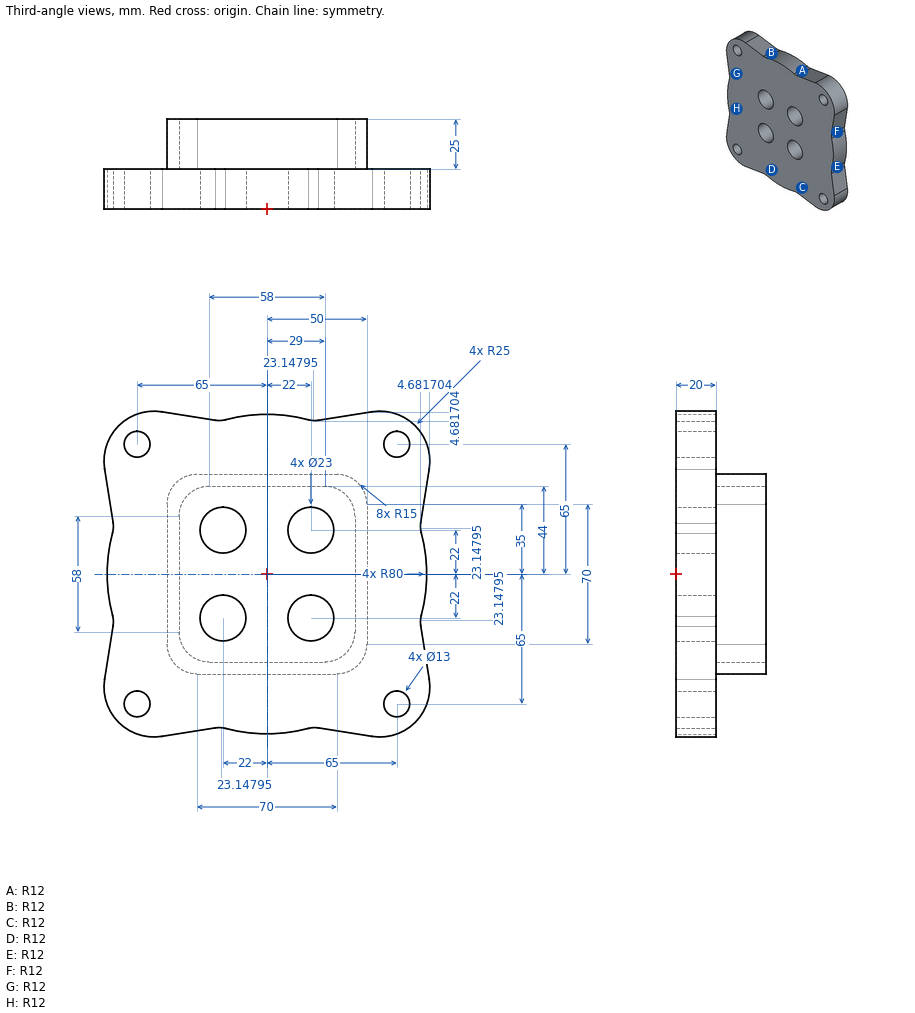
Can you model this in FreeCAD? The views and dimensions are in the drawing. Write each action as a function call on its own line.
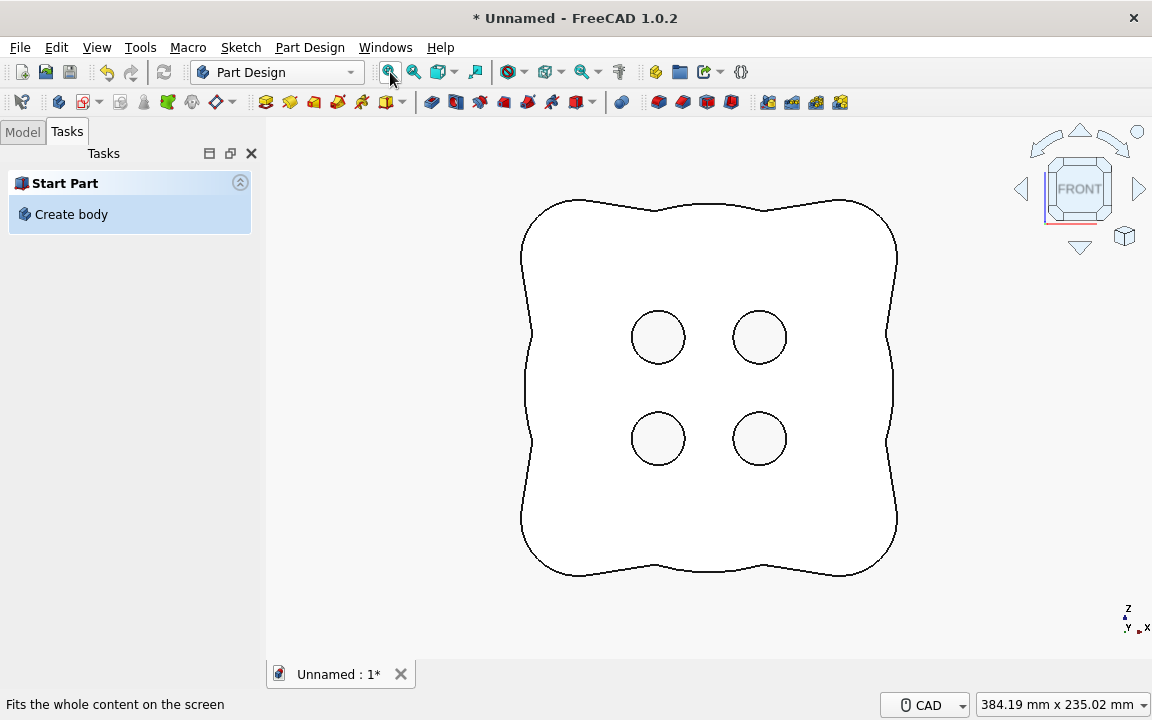
key(3)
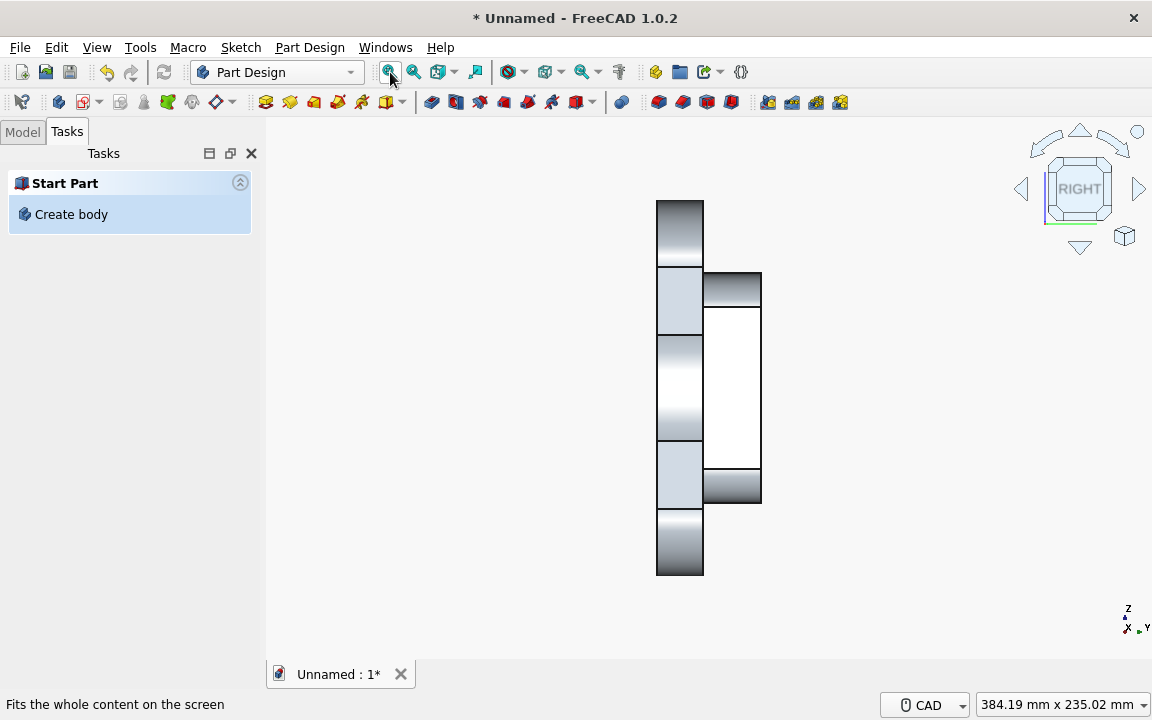
key(5)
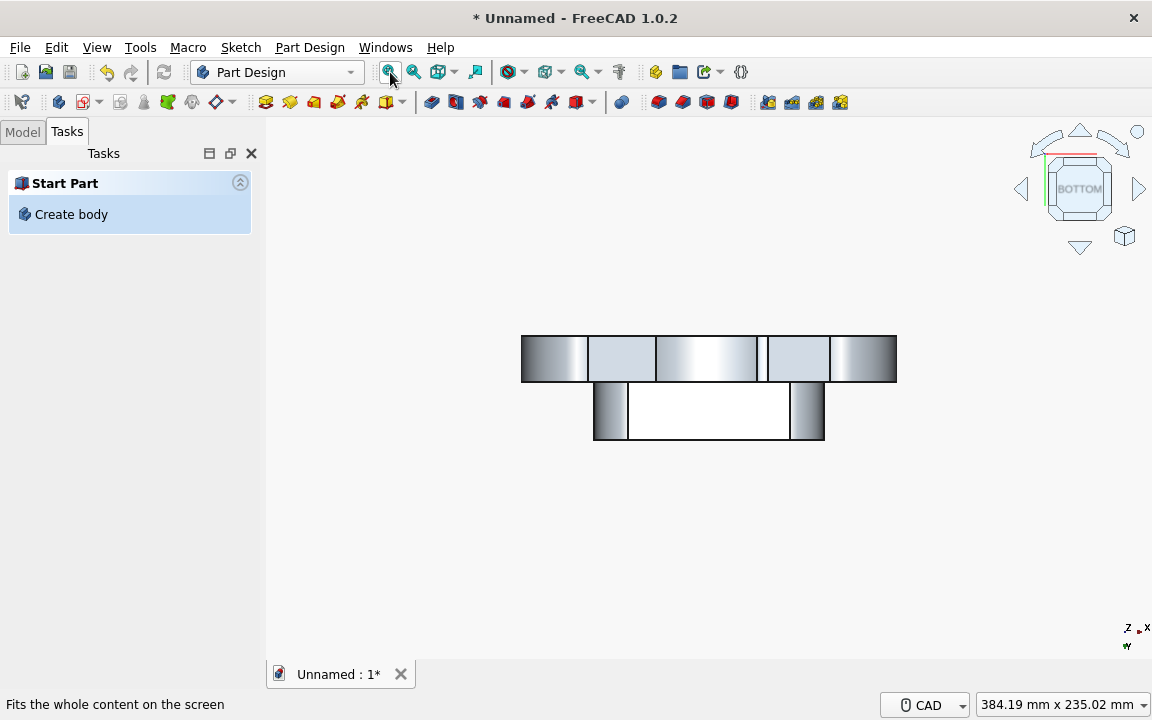
click(390, 72)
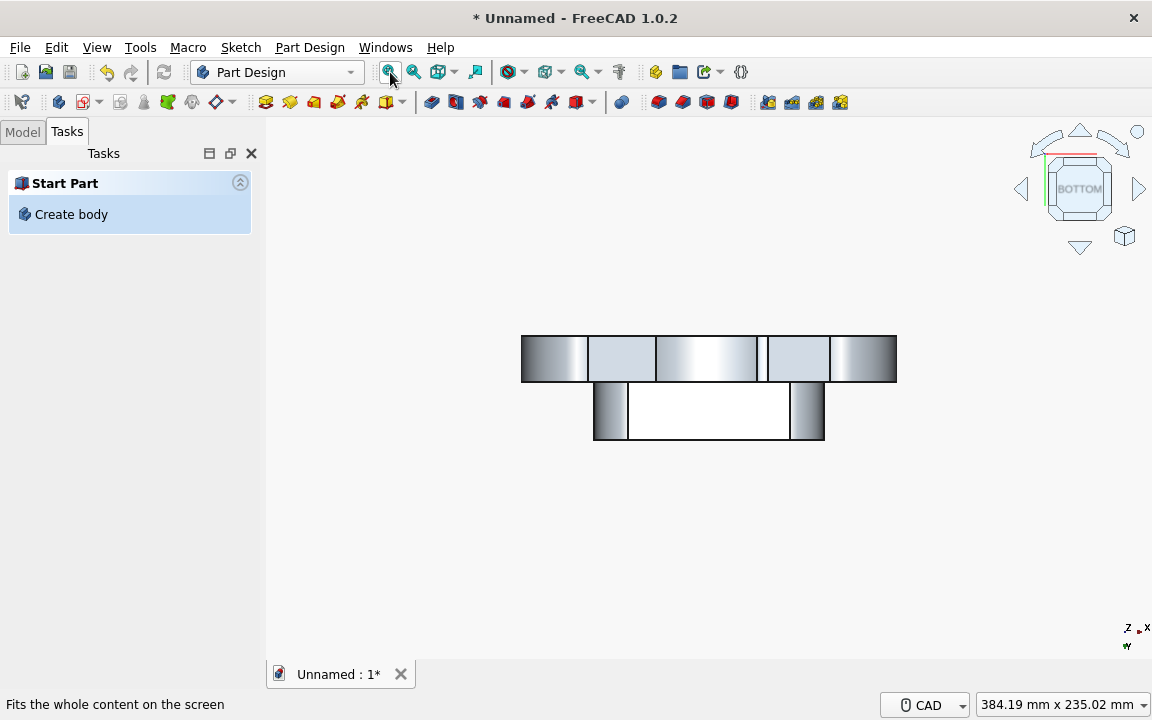
key(4)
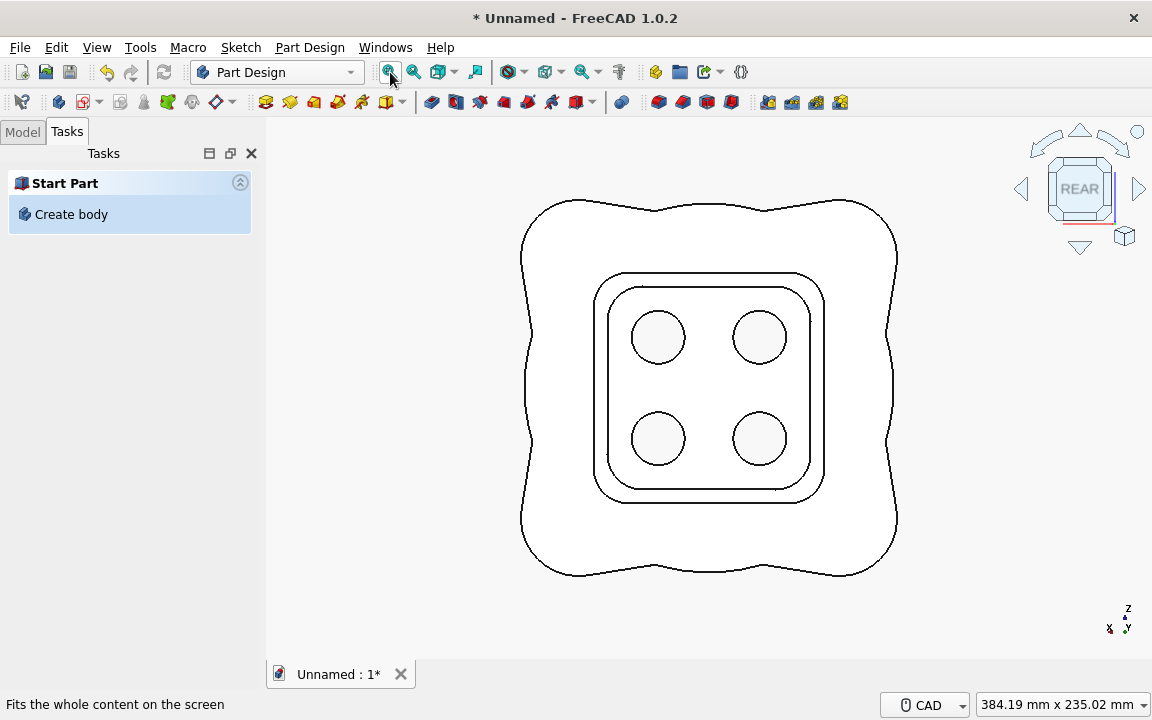
key(6)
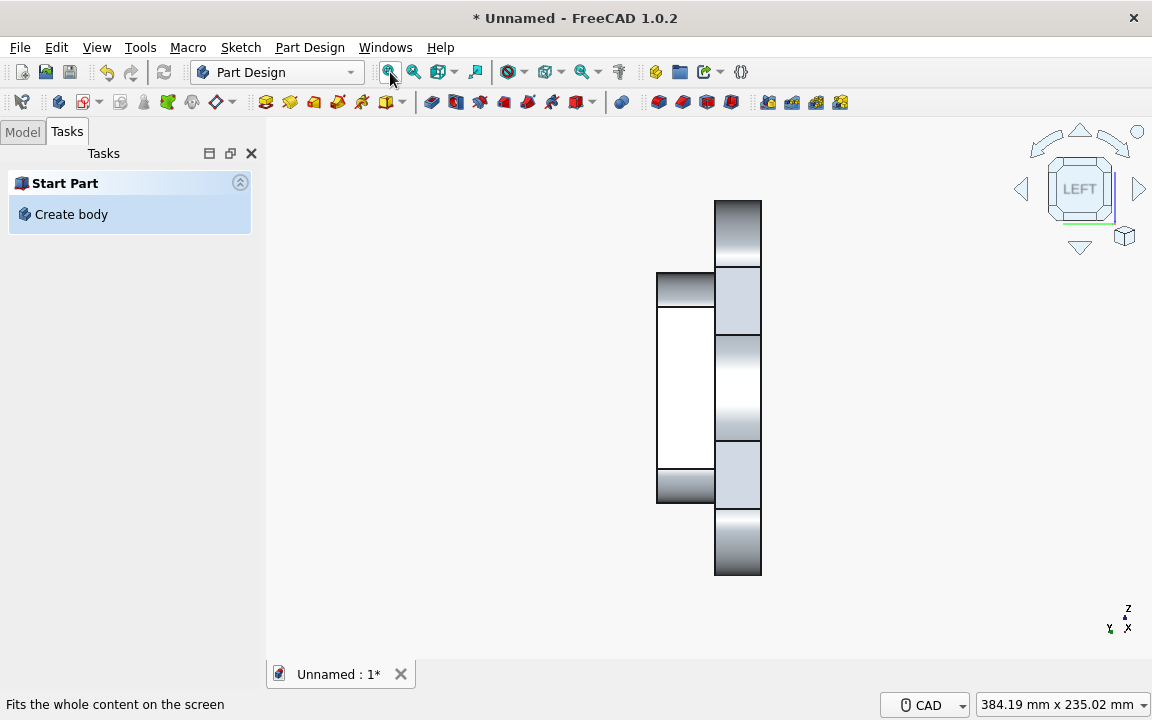
key(v)
key(3)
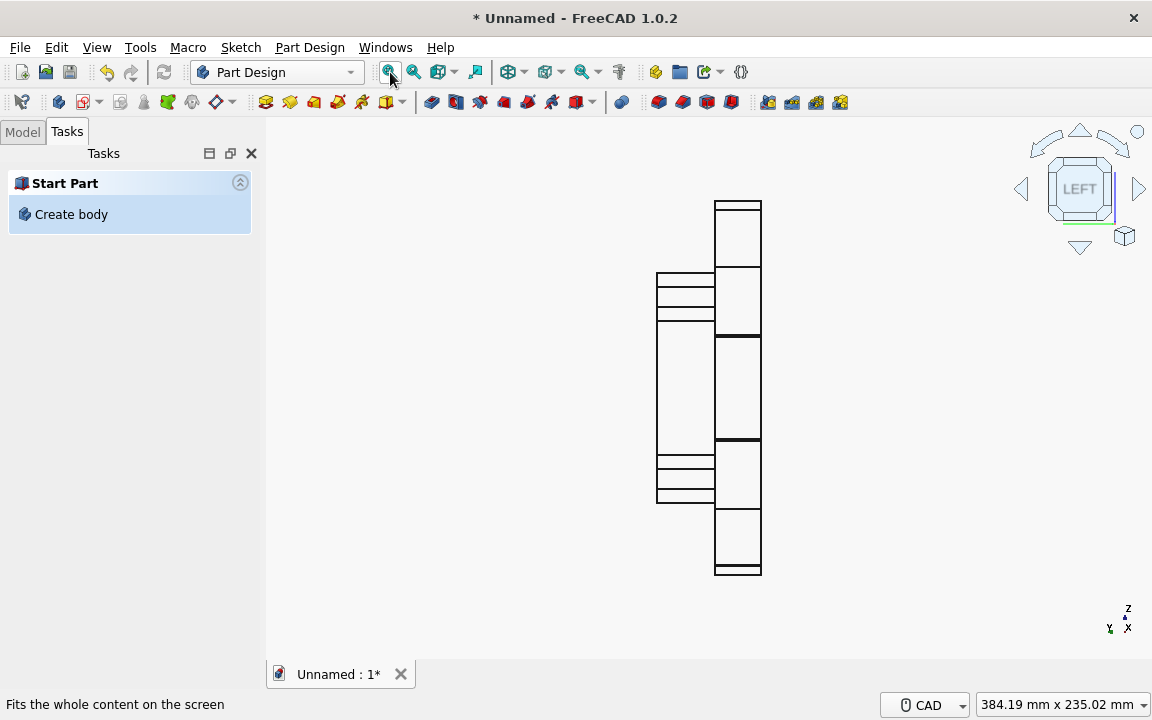
key(0)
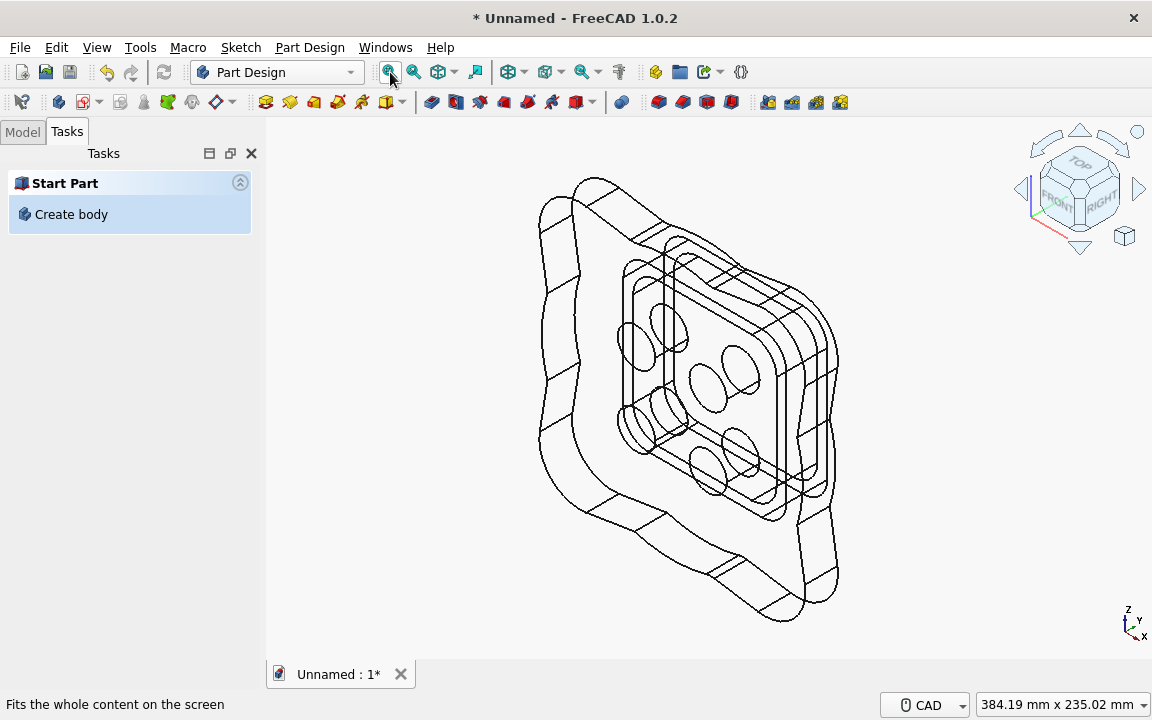
click(651, 521)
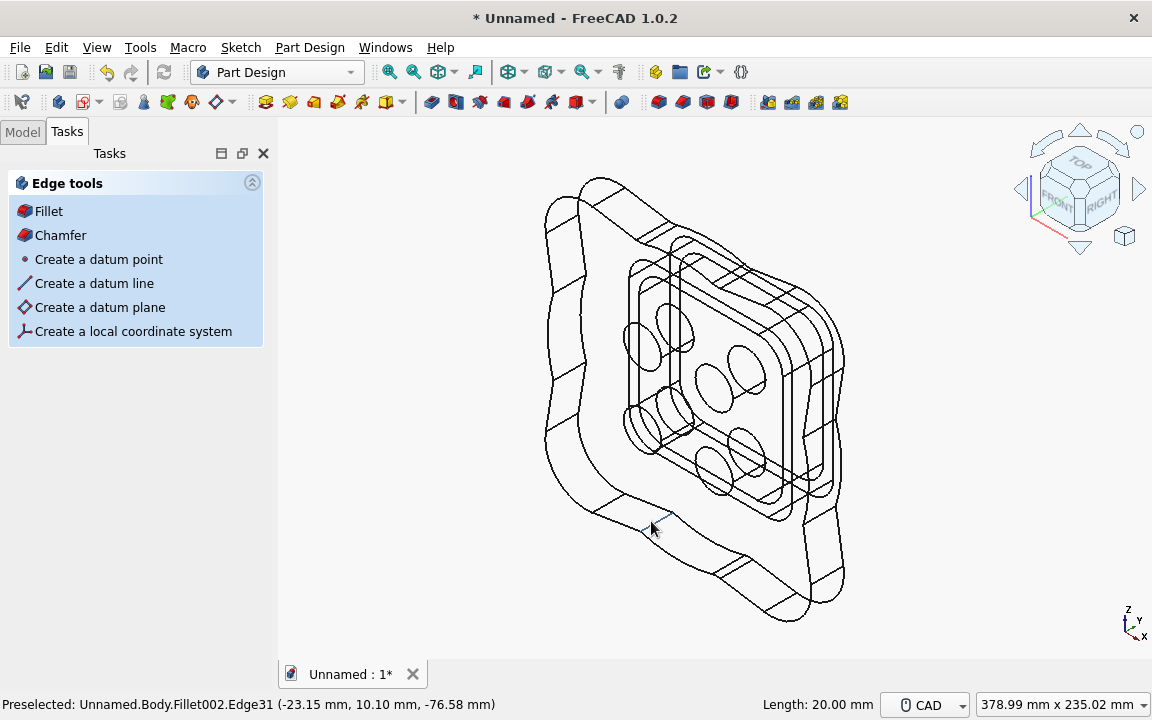
key(v)
key(1)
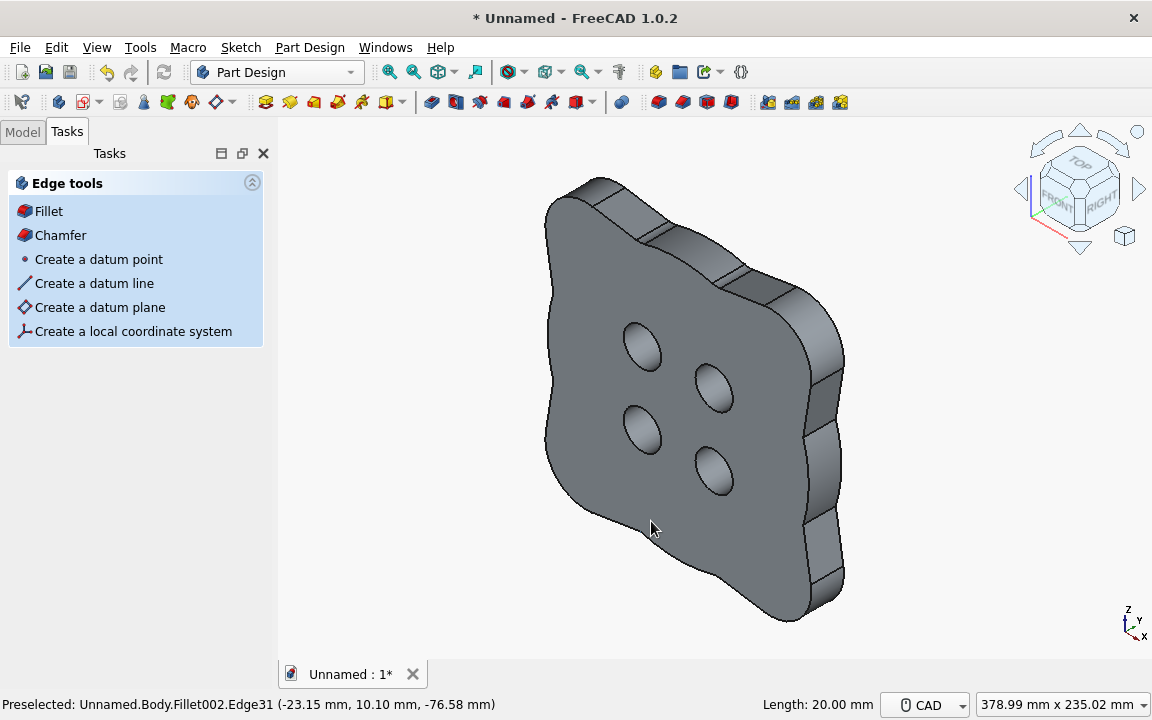
click(660, 102)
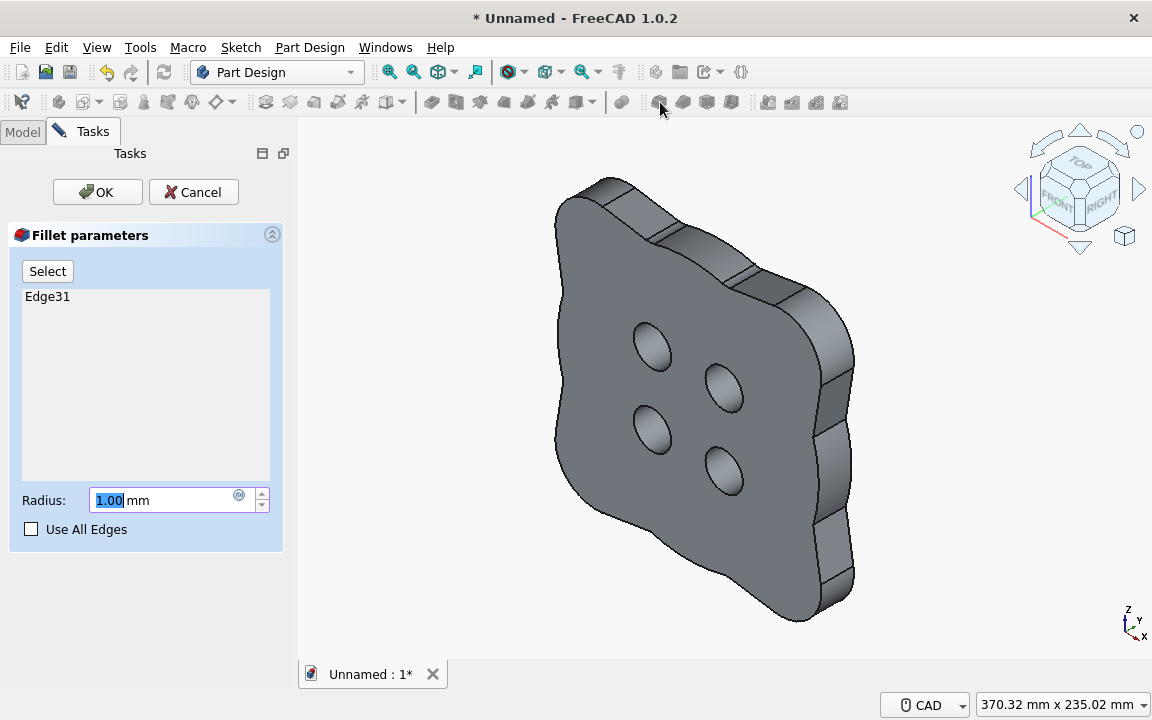
text(12)
key(Tab)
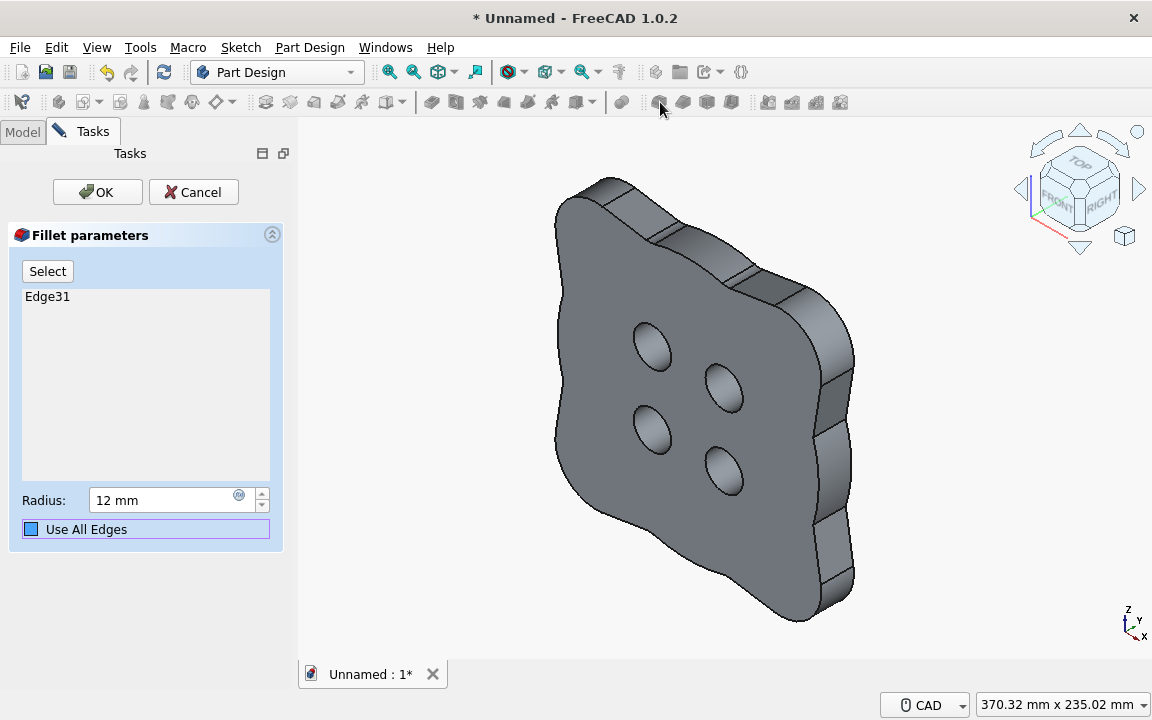
click(98, 192)